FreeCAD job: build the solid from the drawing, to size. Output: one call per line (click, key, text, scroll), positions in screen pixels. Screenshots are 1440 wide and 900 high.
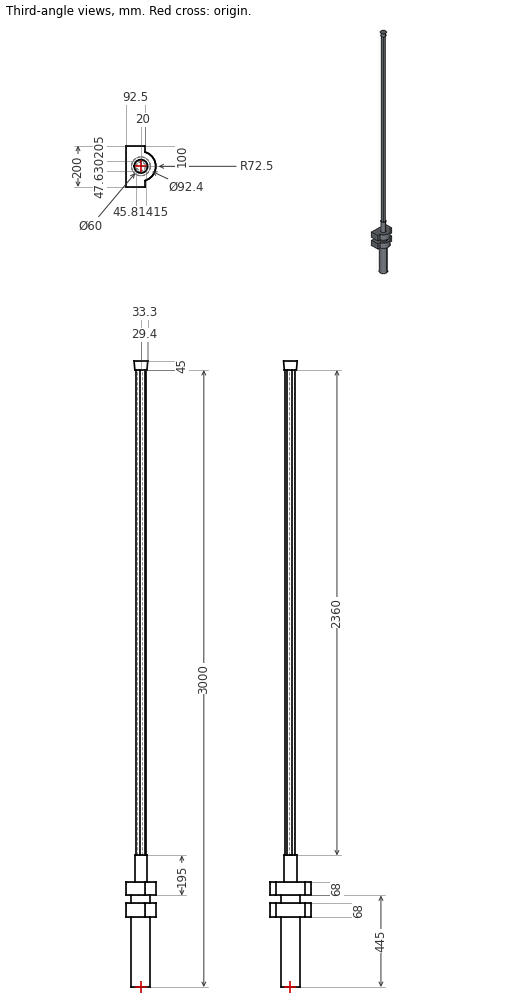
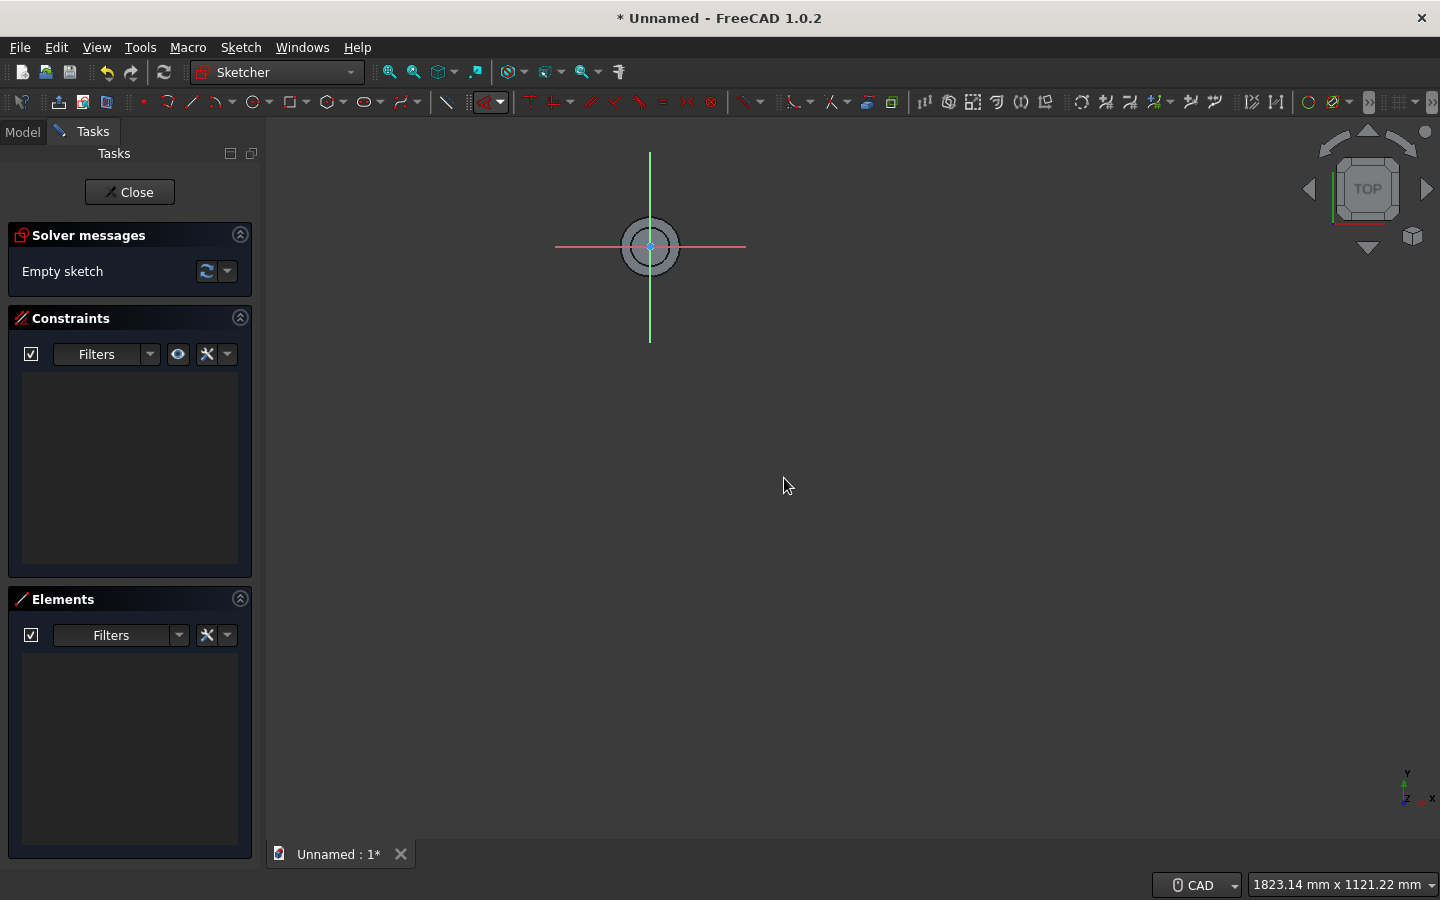
scroll(592, 147, up, 6)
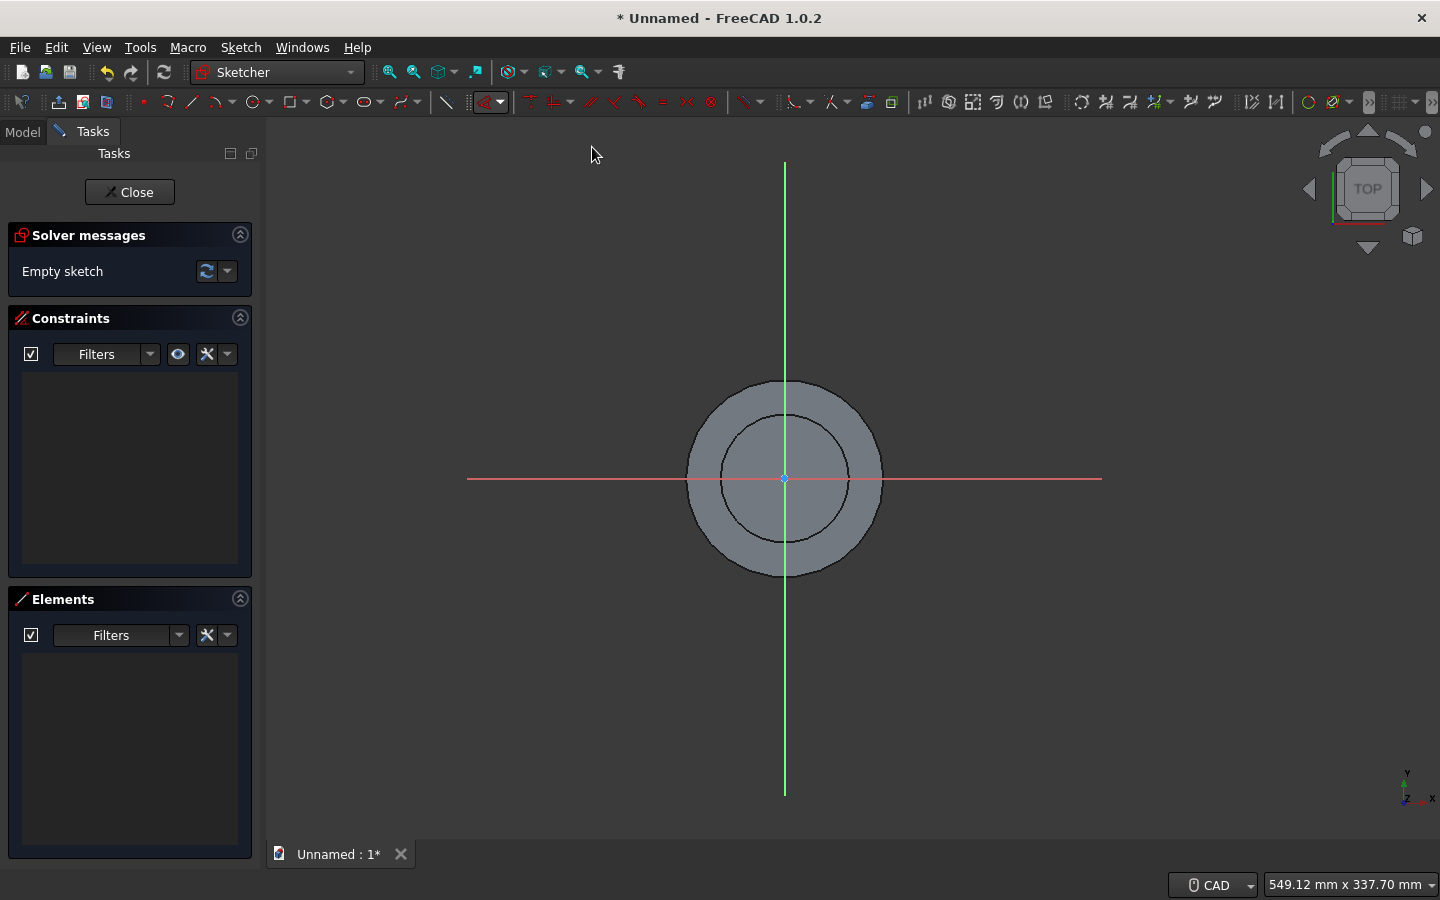
key(g)
key(m)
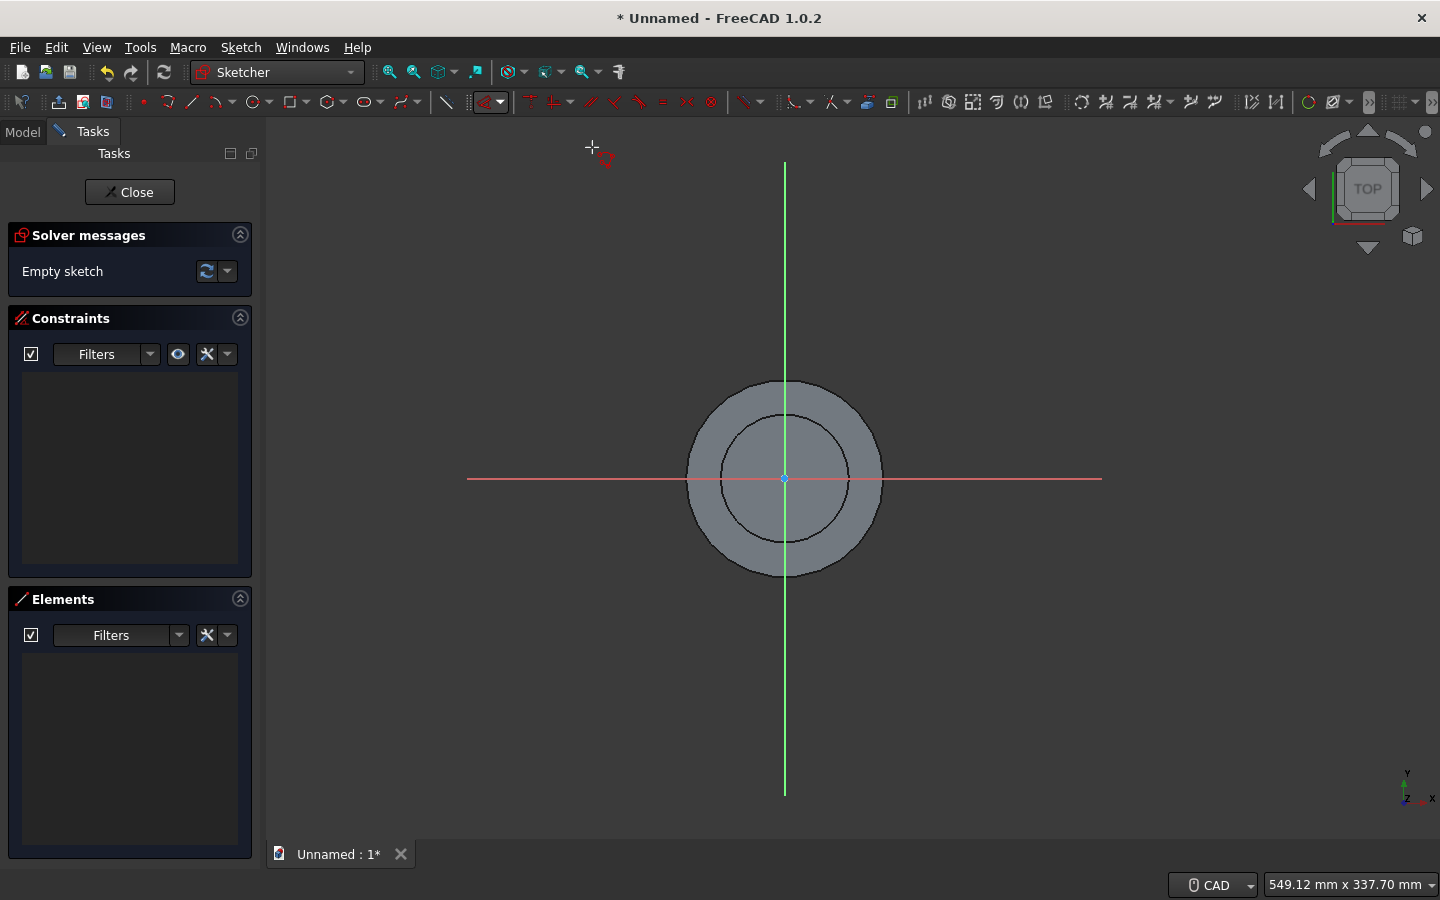
click(827, 330)
click(827, 265)
click(630, 265)
click(630, 692)
click(827, 692)
click(827, 628)
right_click(827, 628)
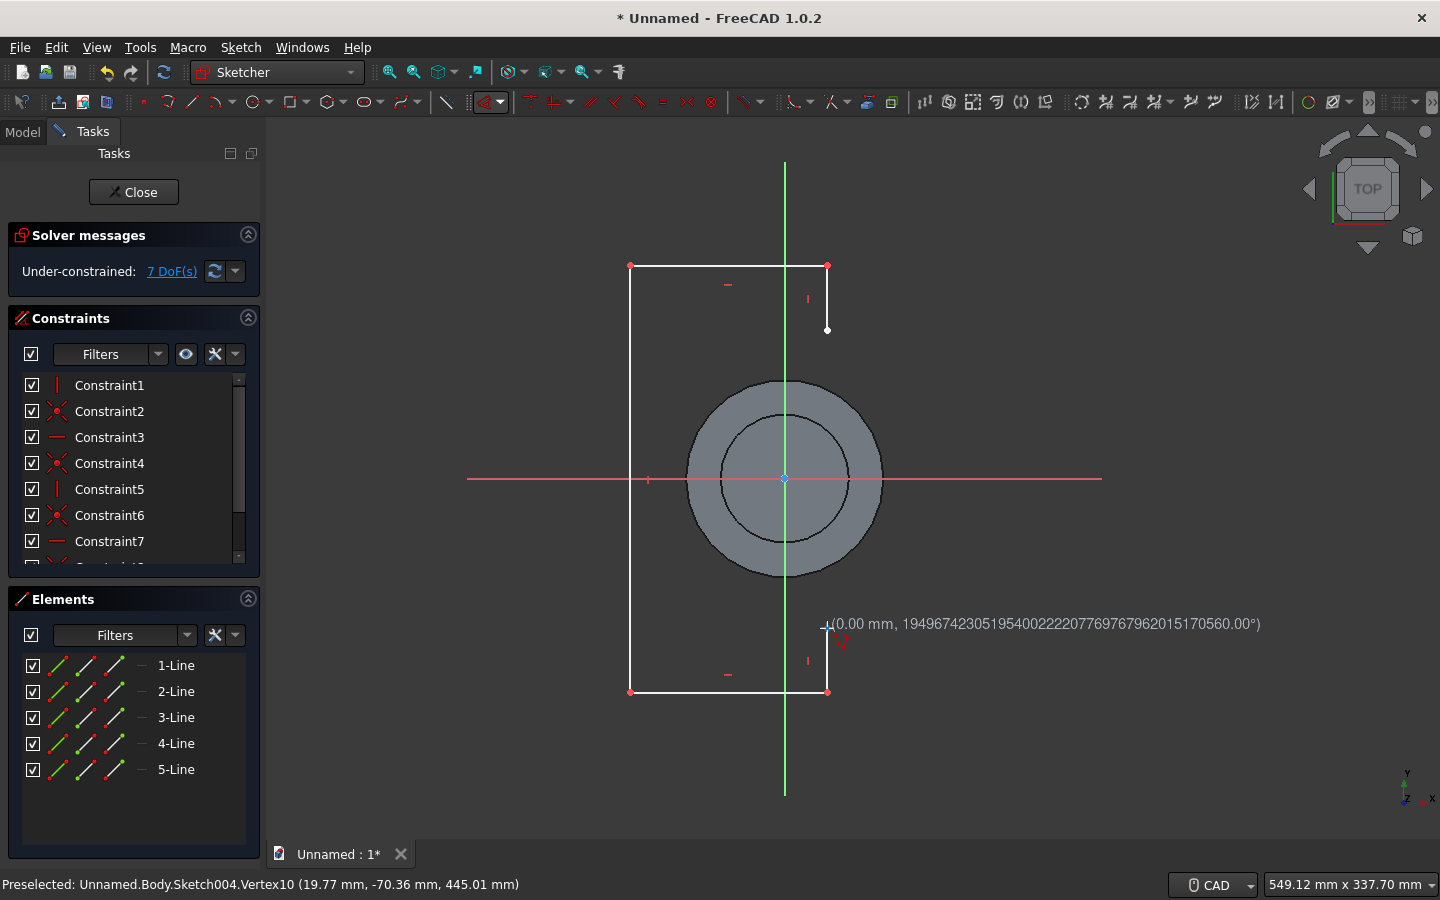
key(g)
key(3)
key(a)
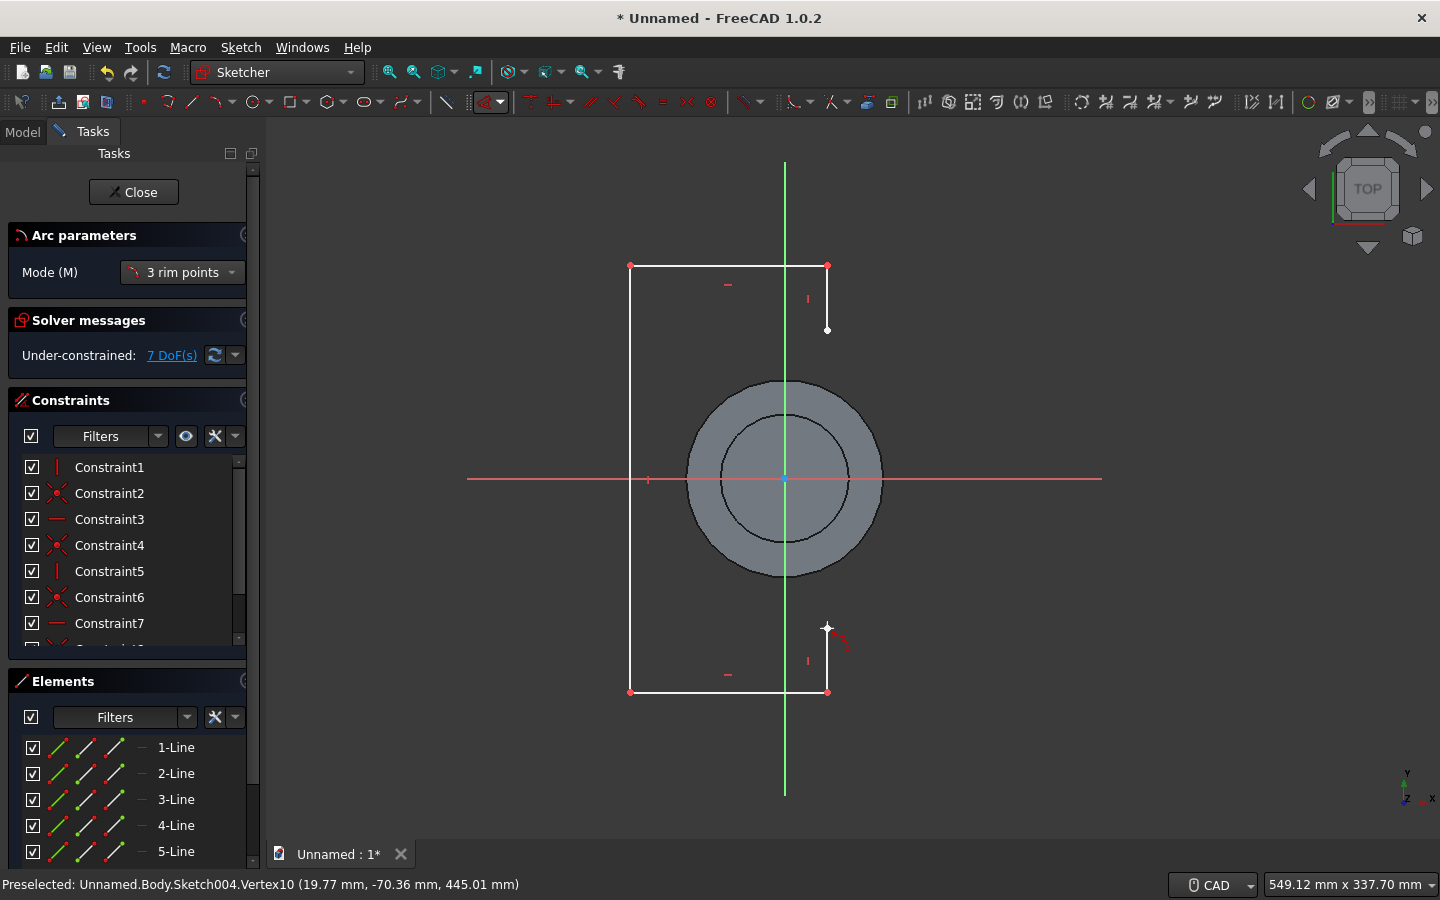
click(827, 629)
click(827, 331)
click(935, 518)
key(Escape)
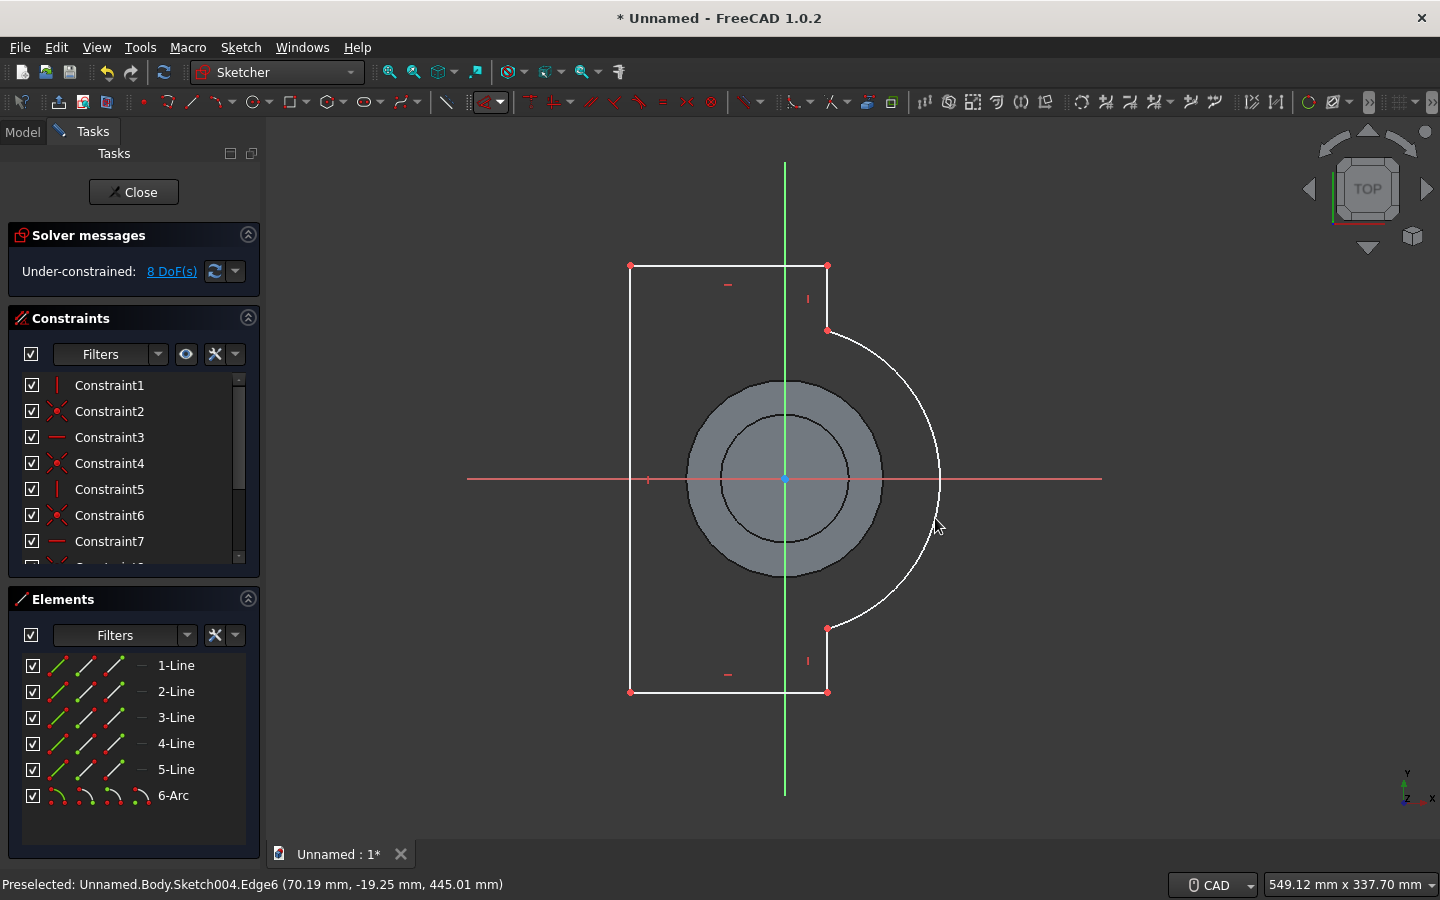
drag(775, 469, 795, 490)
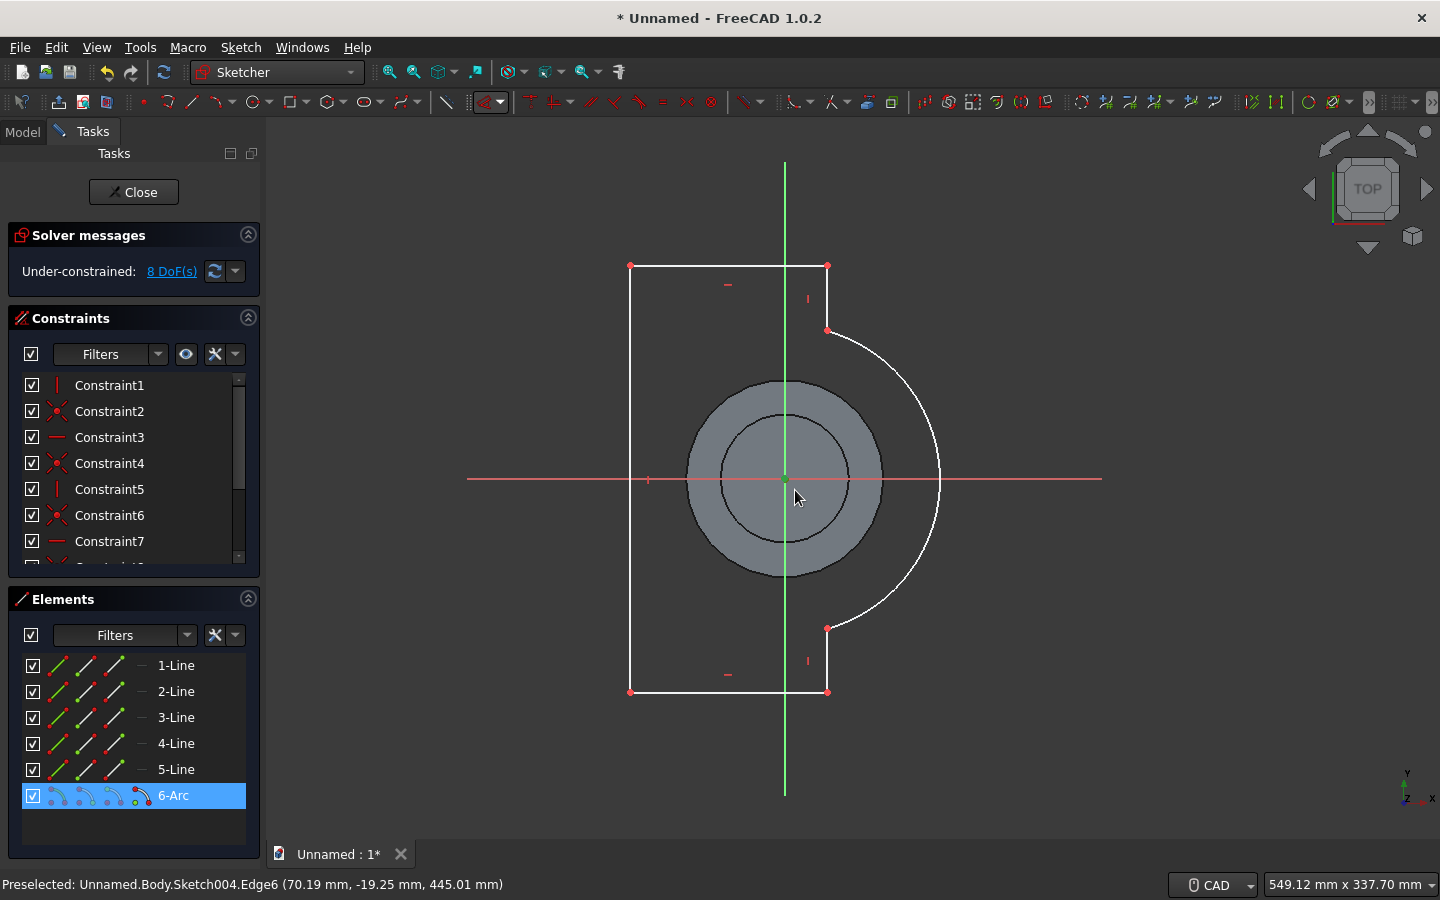
key(c)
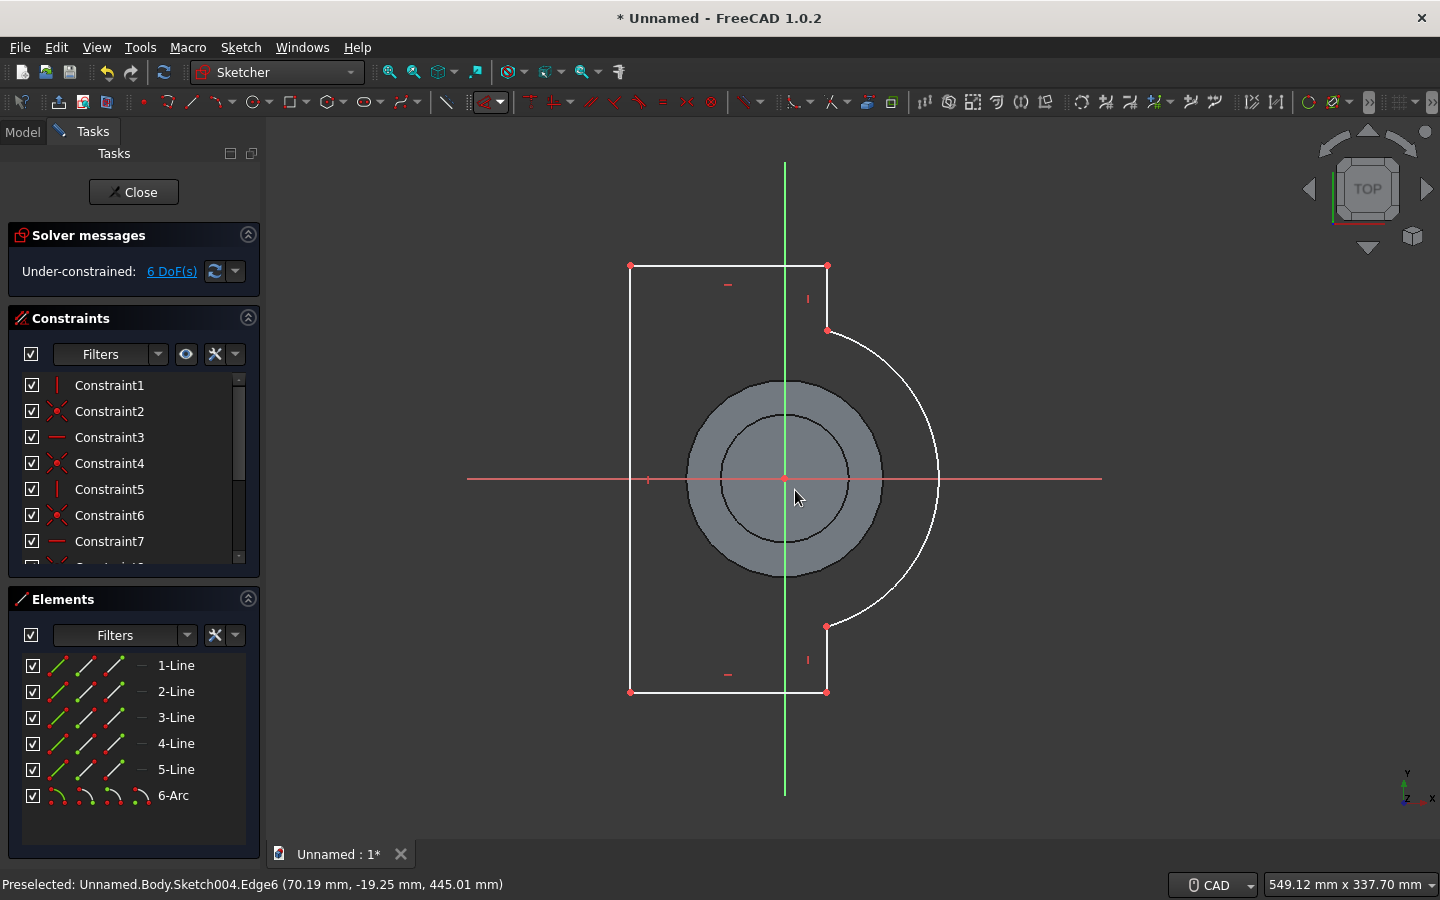
click(919, 555)